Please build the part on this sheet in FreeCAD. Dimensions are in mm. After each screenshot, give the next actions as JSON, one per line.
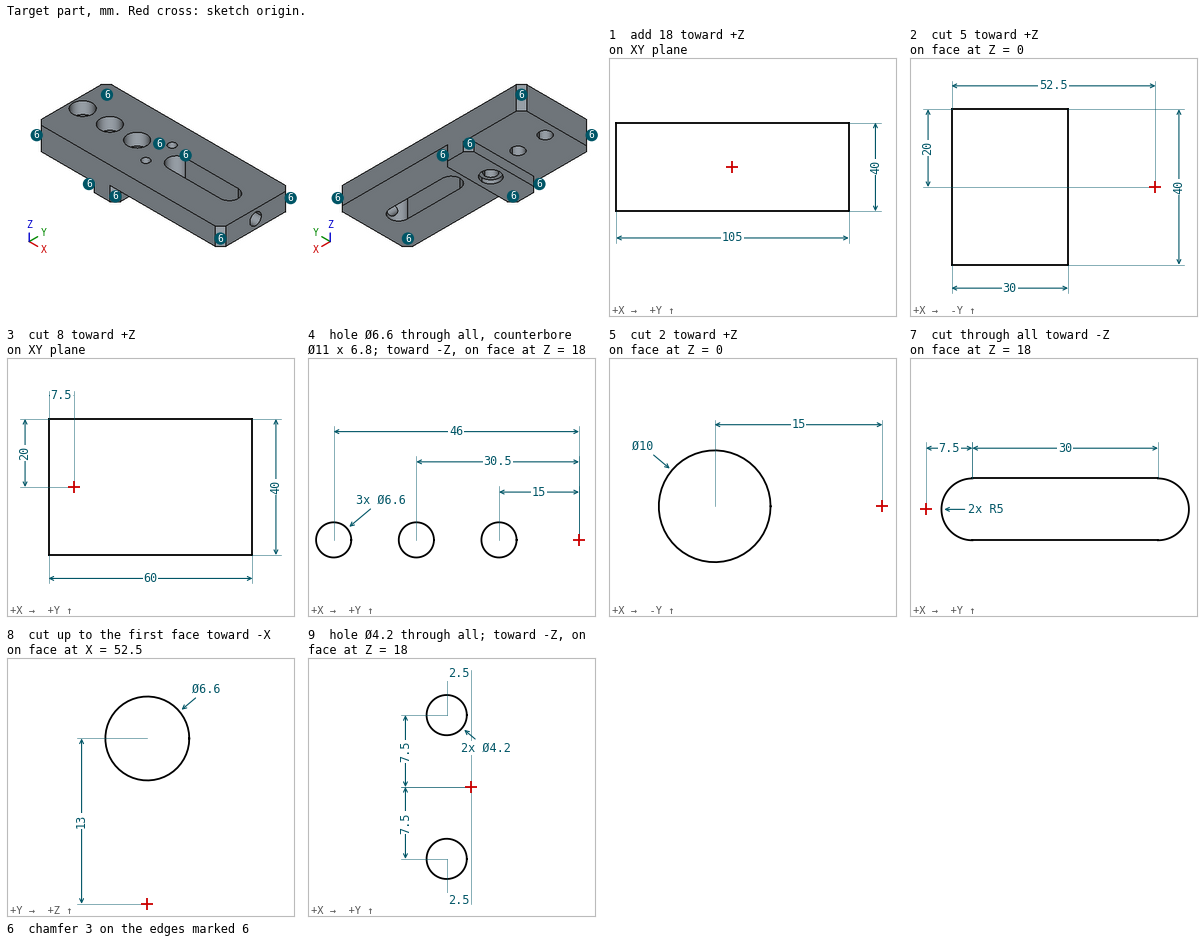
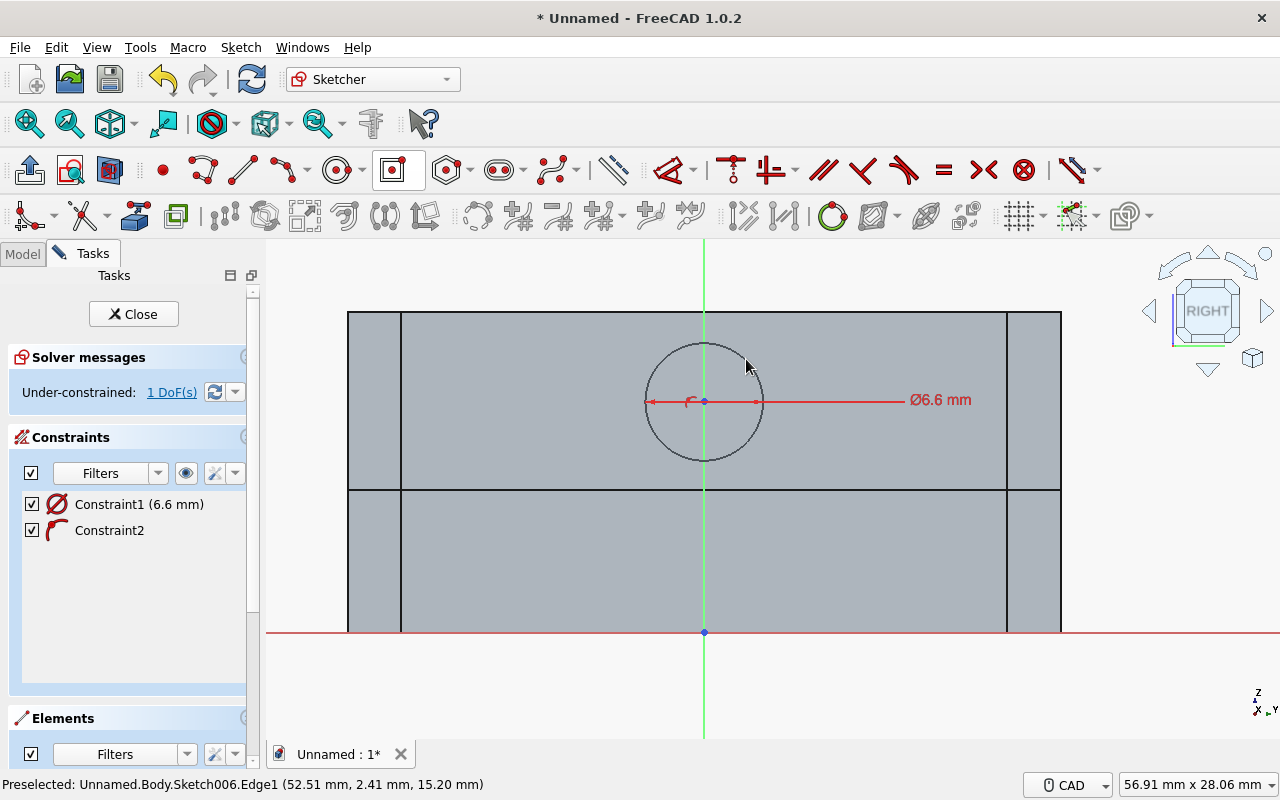
{"action": "key", "text": "d"}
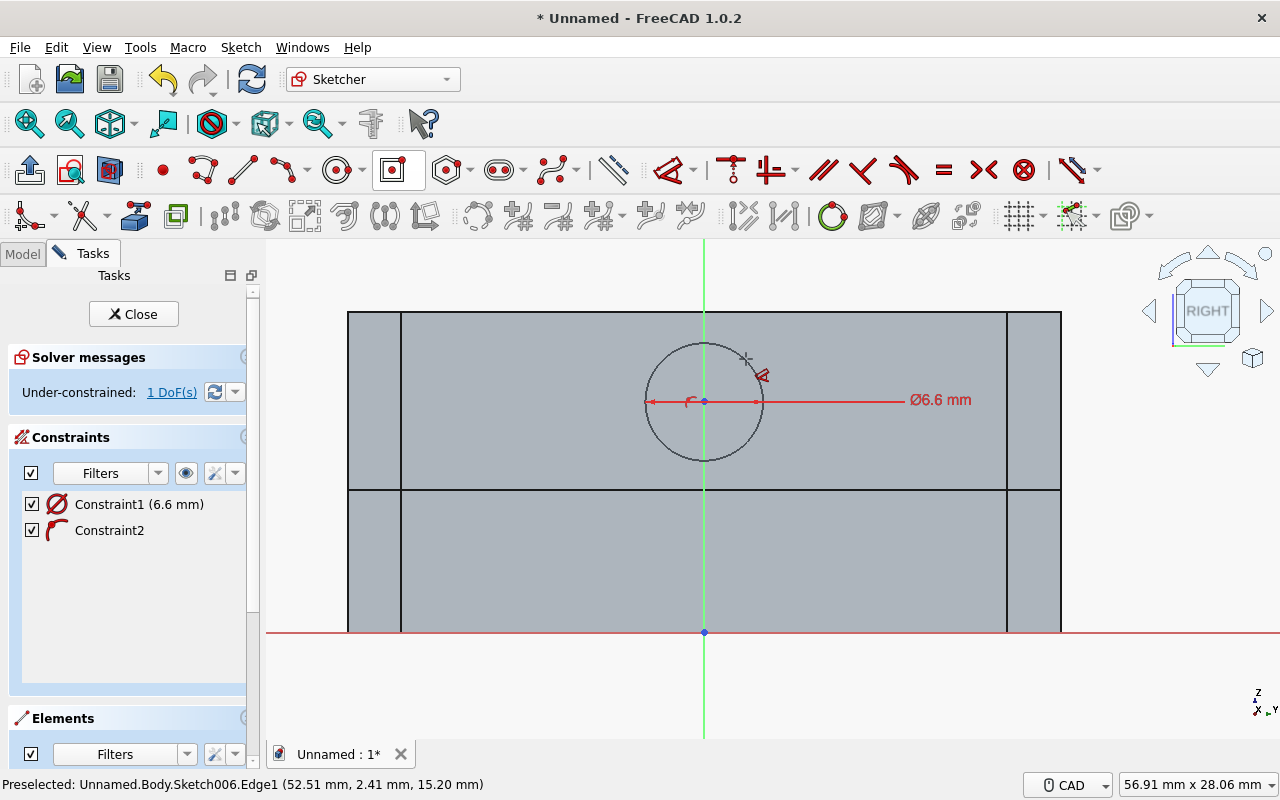
{"action": "left_click", "coordinate": [704, 402]}
{"action": "left_click", "coordinate": [738, 517]}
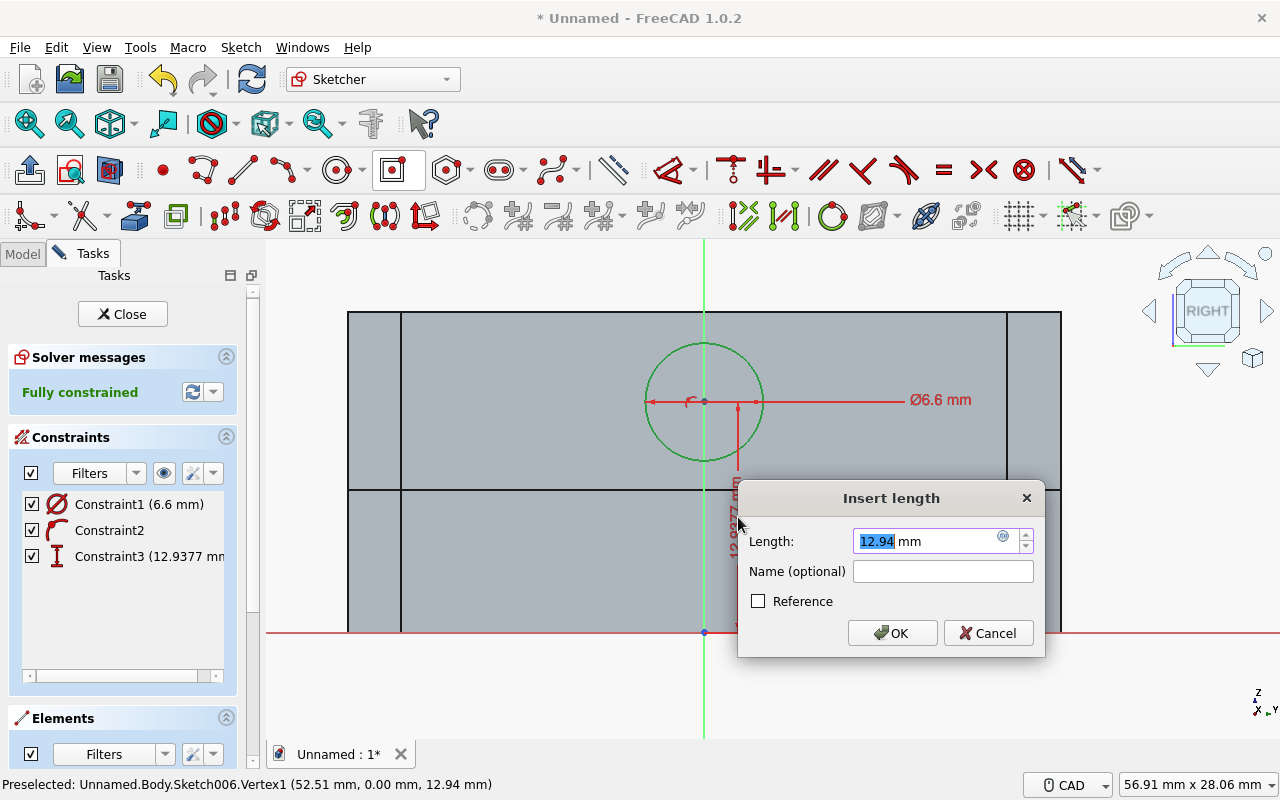
{"action": "type", "text": "13"}
{"action": "key", "text": "Return"}
{"action": "key", "text": "Escape"}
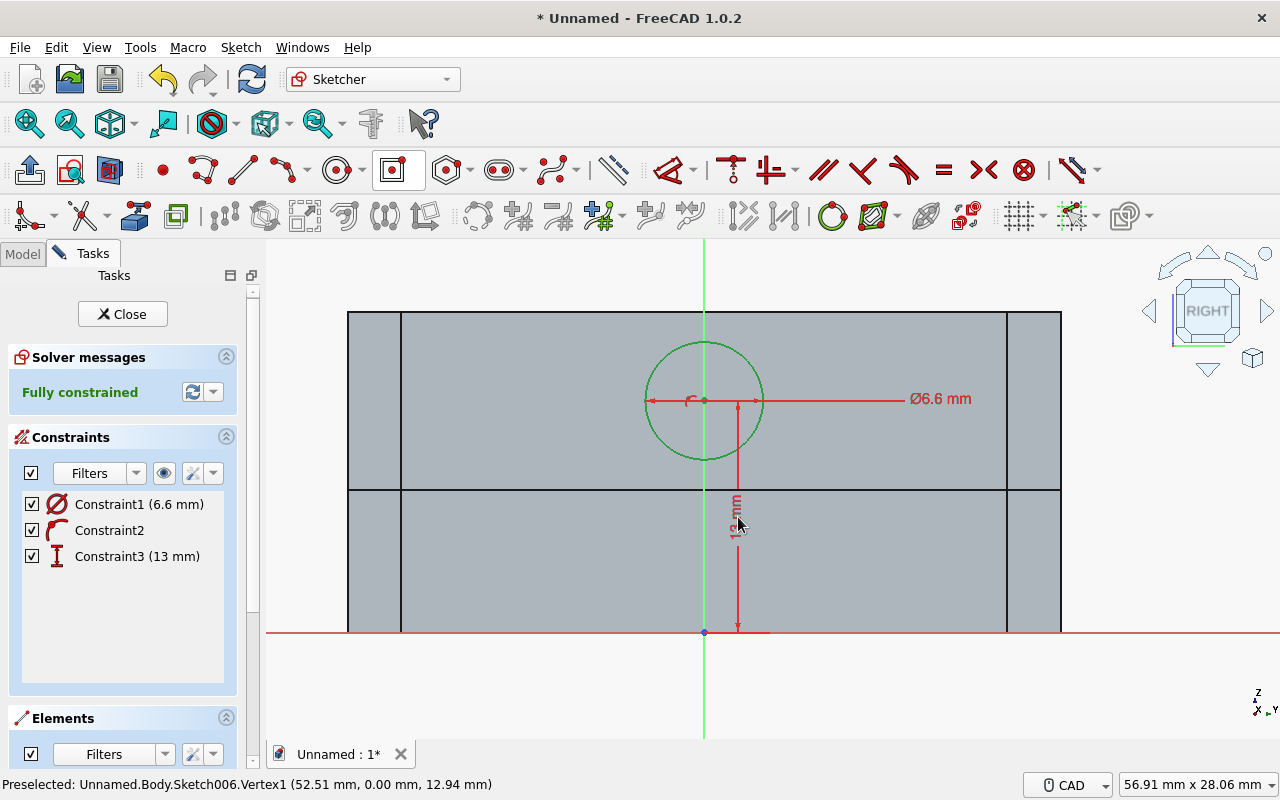
{"action": "left_click", "coordinate": [123, 314]}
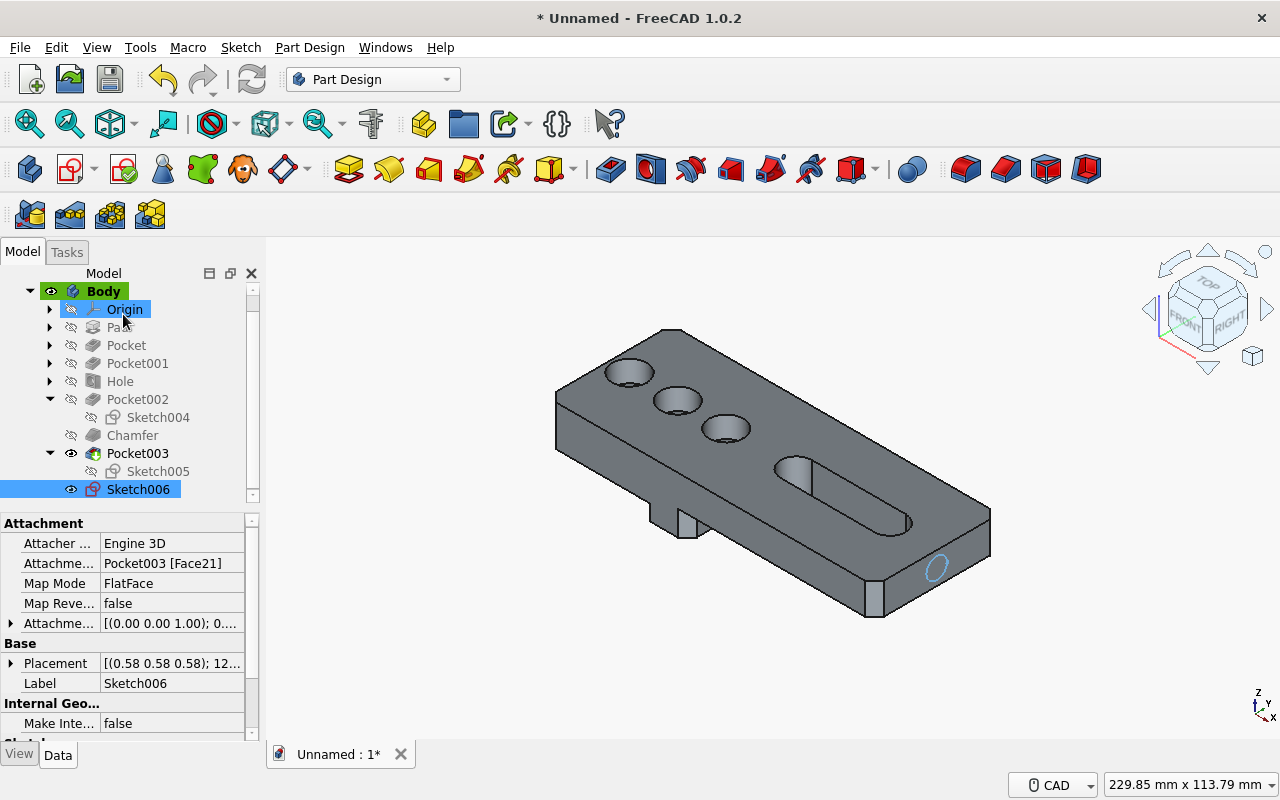
{"action": "left_click", "coordinate": [612, 170]}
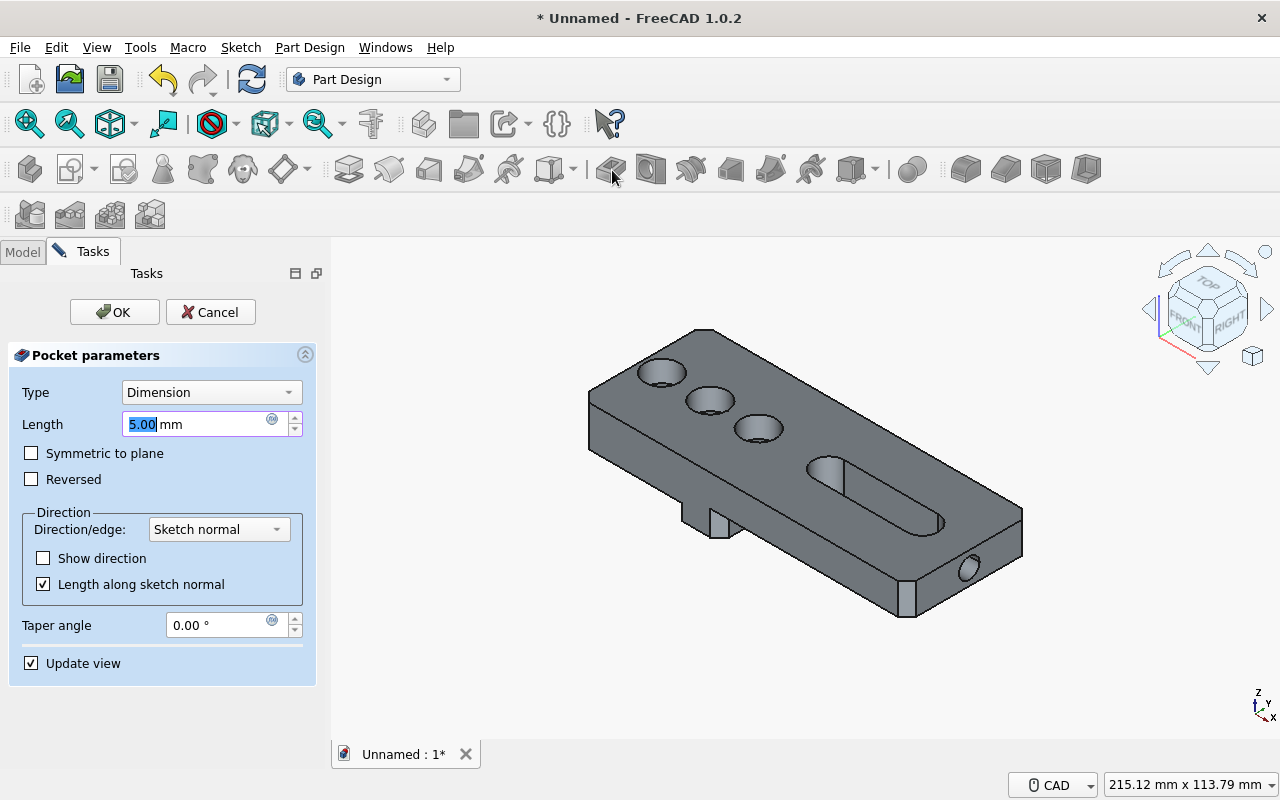
{"action": "left_click", "coordinate": [212, 392]}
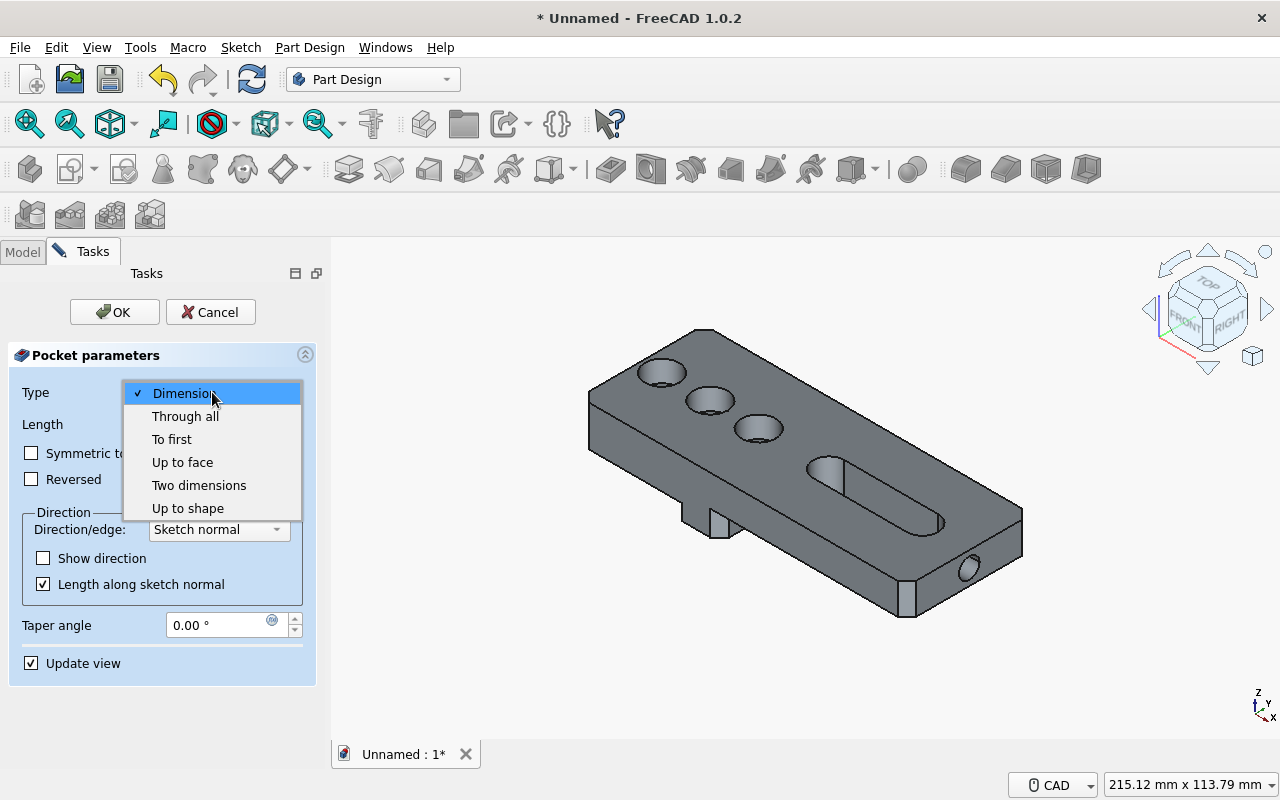
{"action": "left_click", "coordinate": [212, 440]}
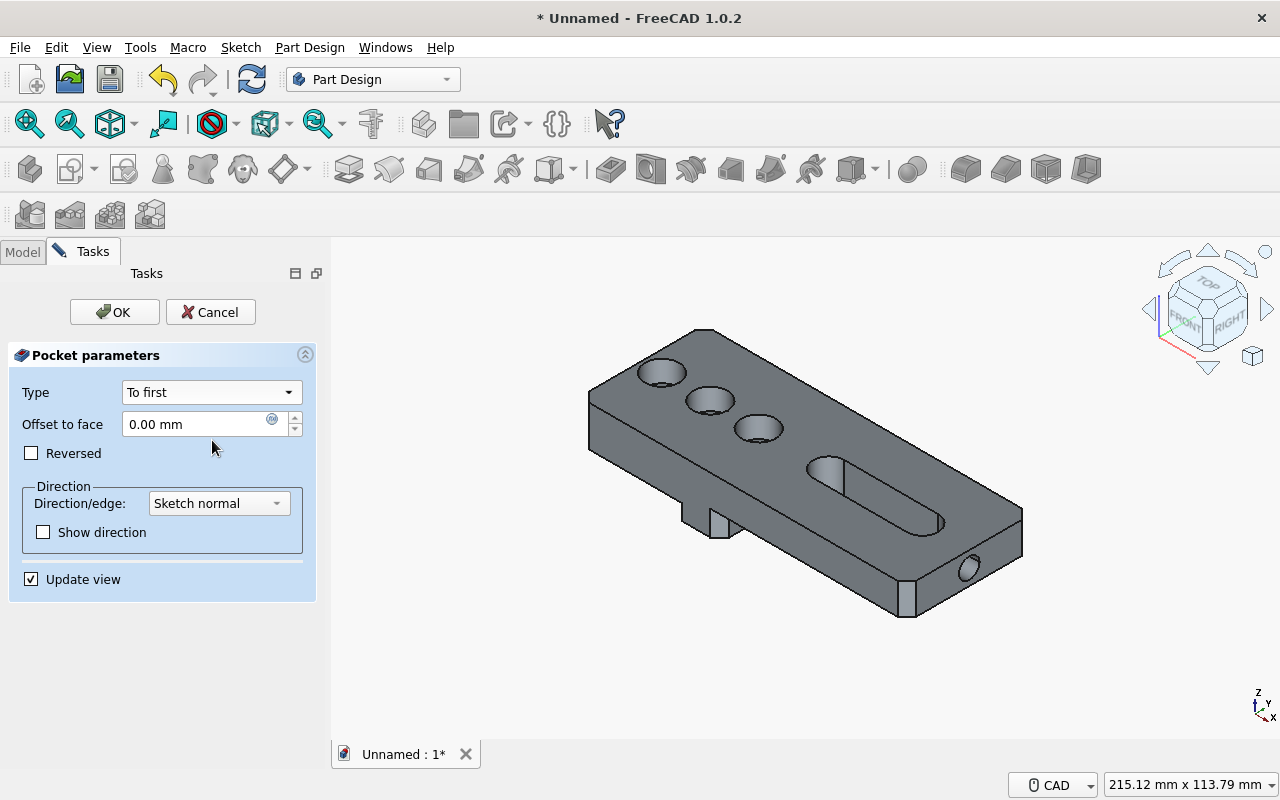
{"action": "left_click", "coordinate": [115, 312]}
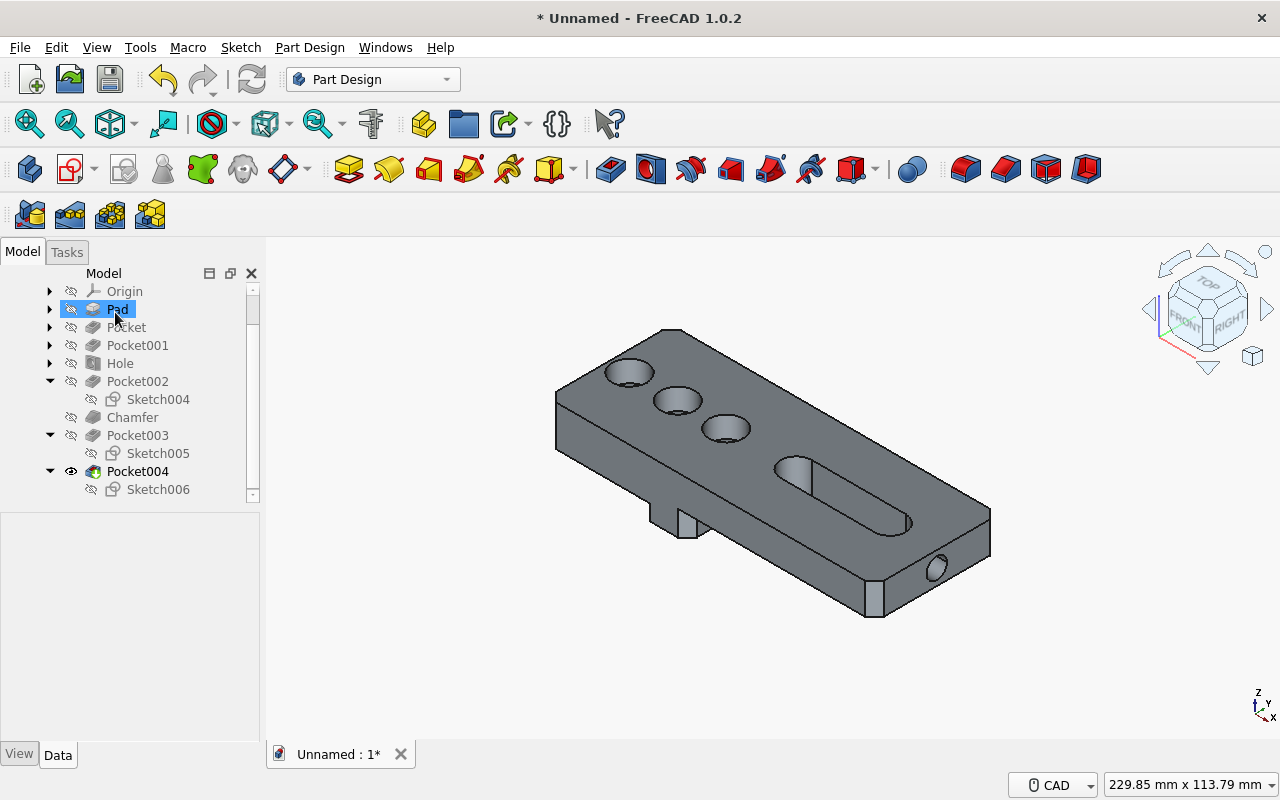
{"action": "left_click", "coordinate": [809, 434]}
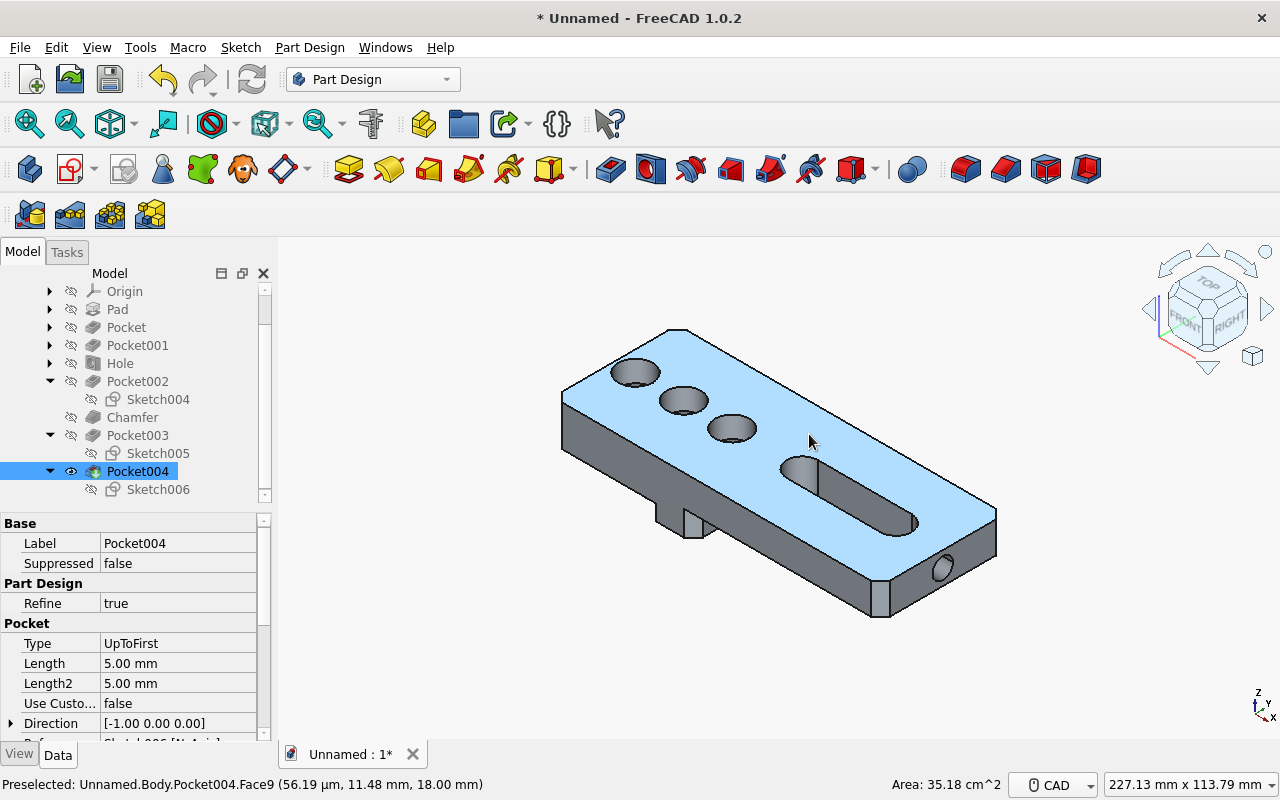
{"action": "left_click", "coordinate": [70, 170]}